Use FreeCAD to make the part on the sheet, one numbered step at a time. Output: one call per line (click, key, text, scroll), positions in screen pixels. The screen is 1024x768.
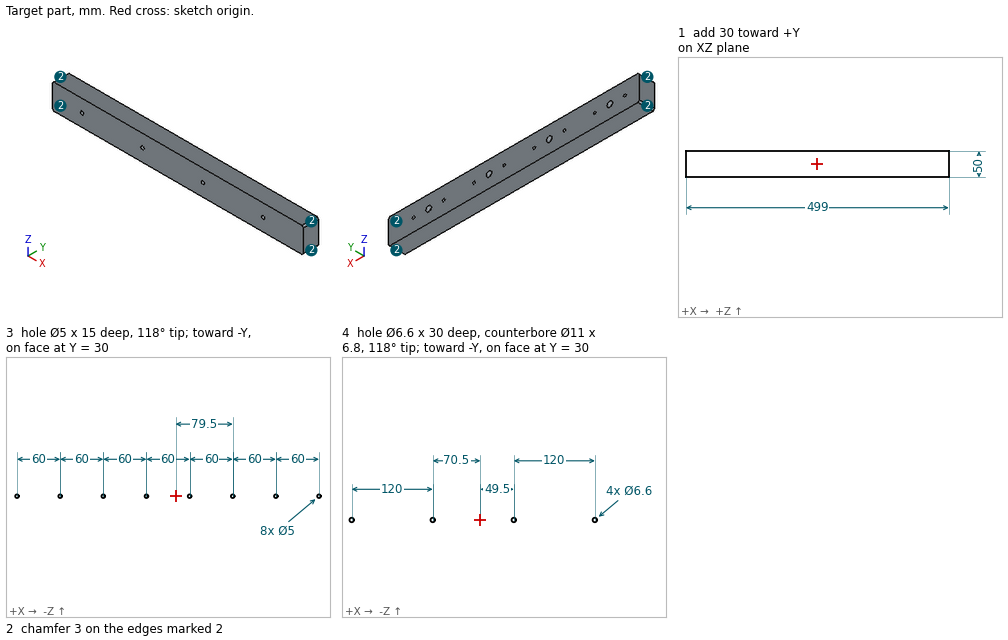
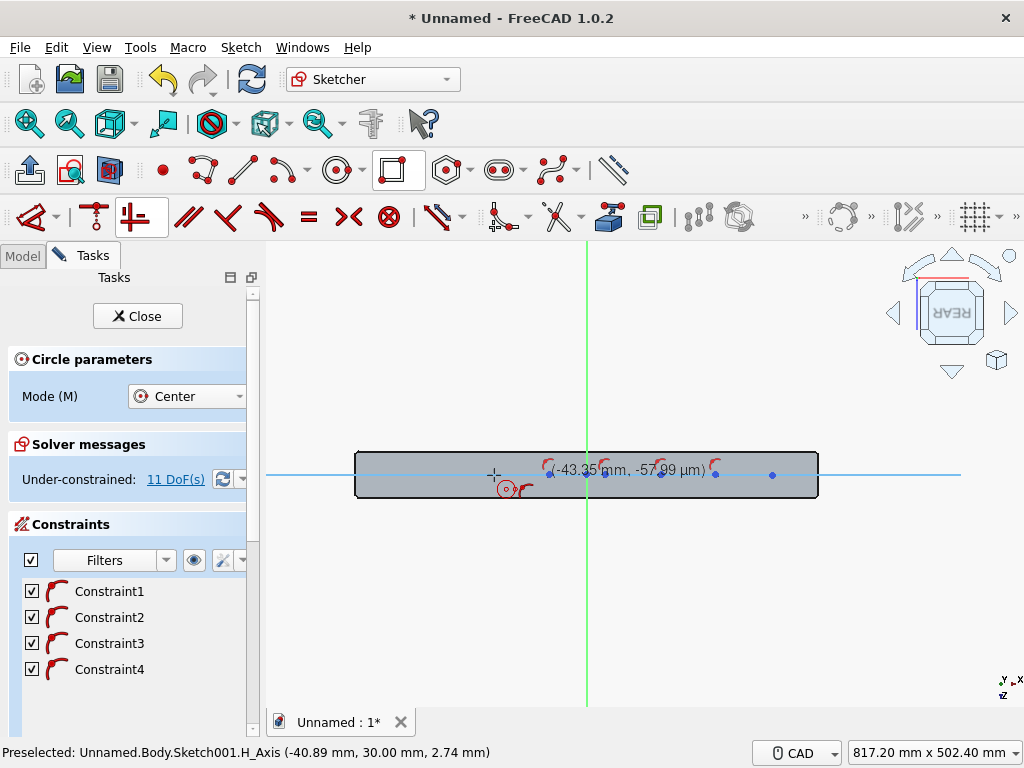
click(494, 475)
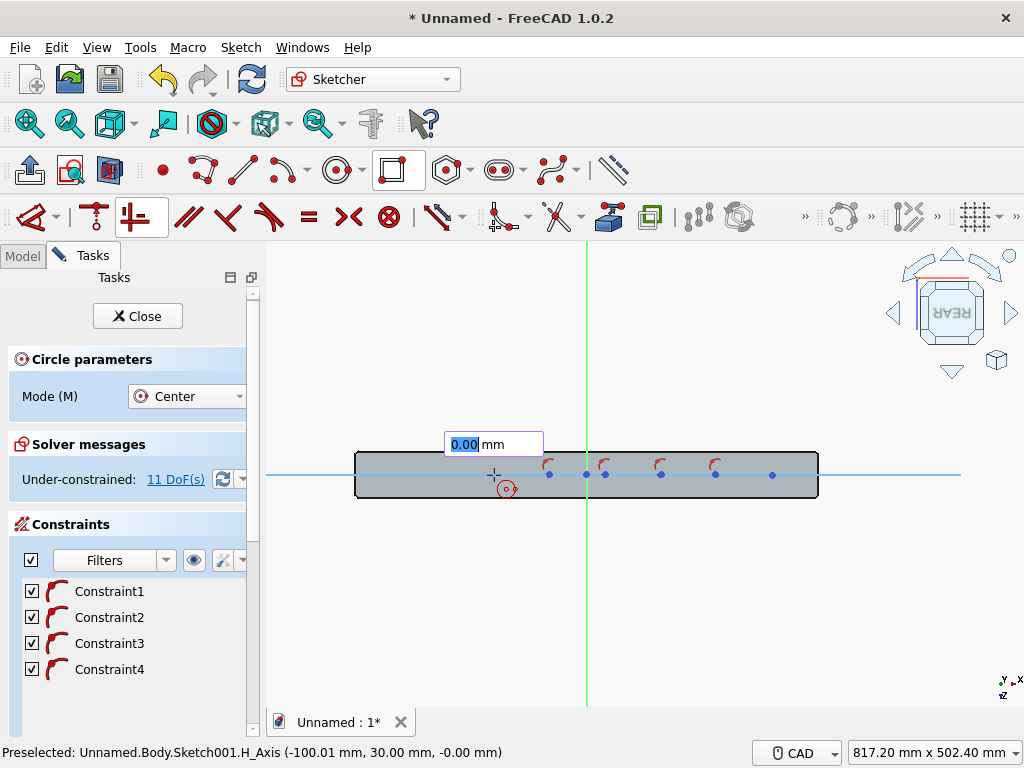
scroll(493, 477, up, 10)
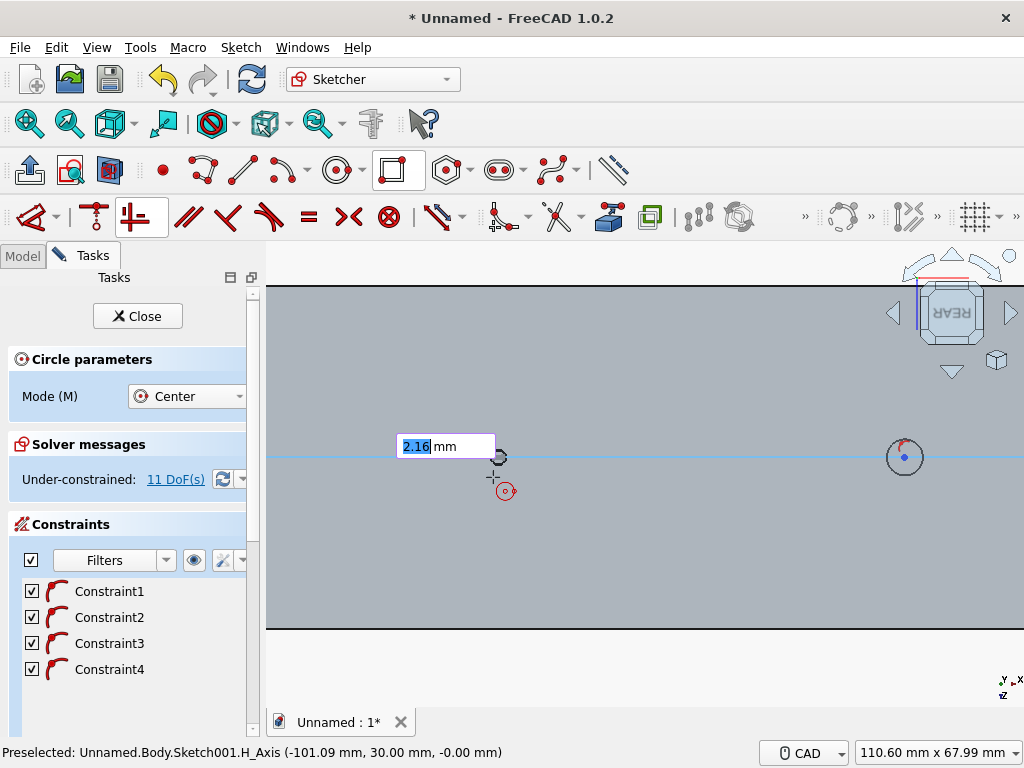
click(489, 474)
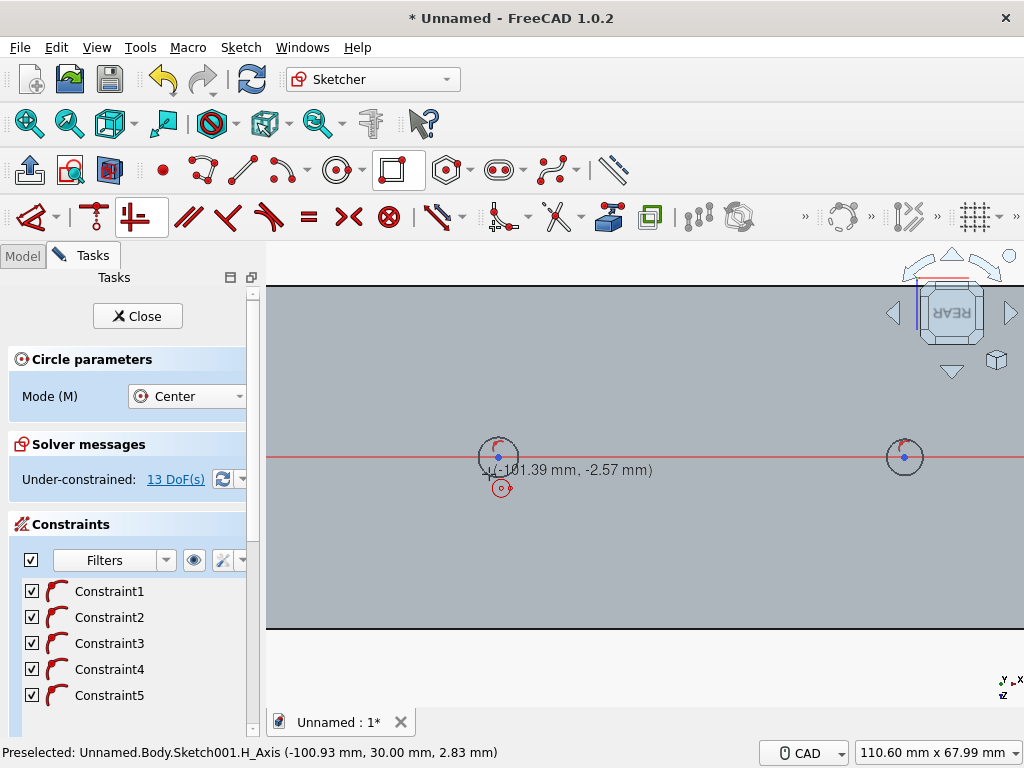
scroll(493, 477, down, 10)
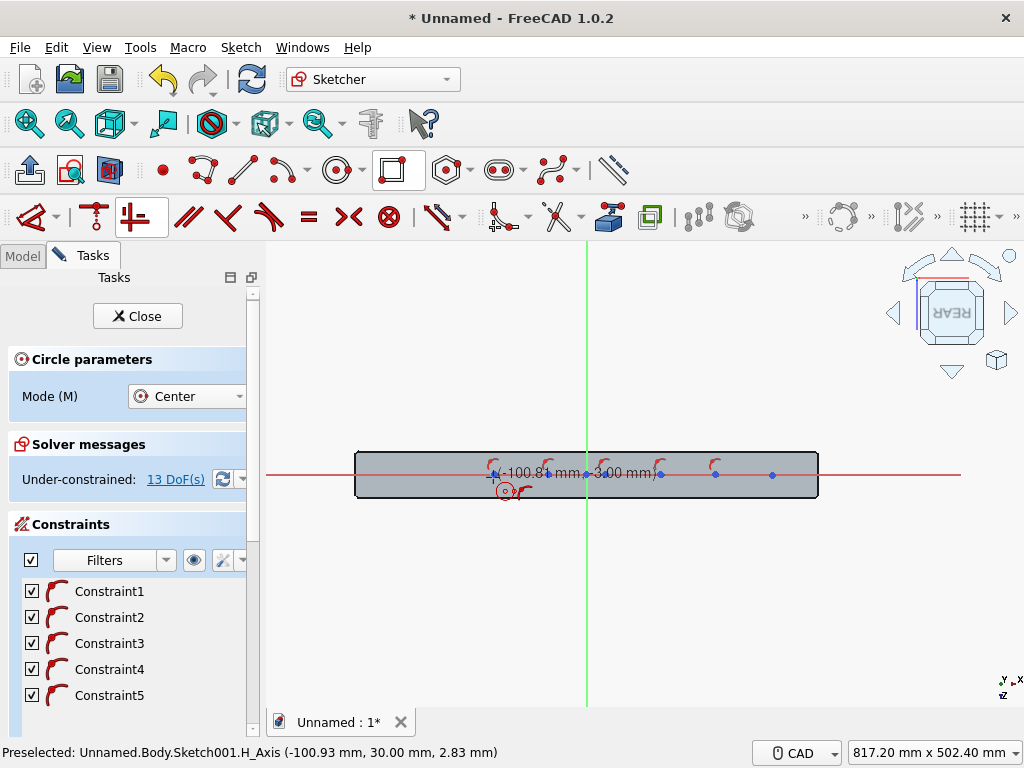
scroll(438, 475, up, 12)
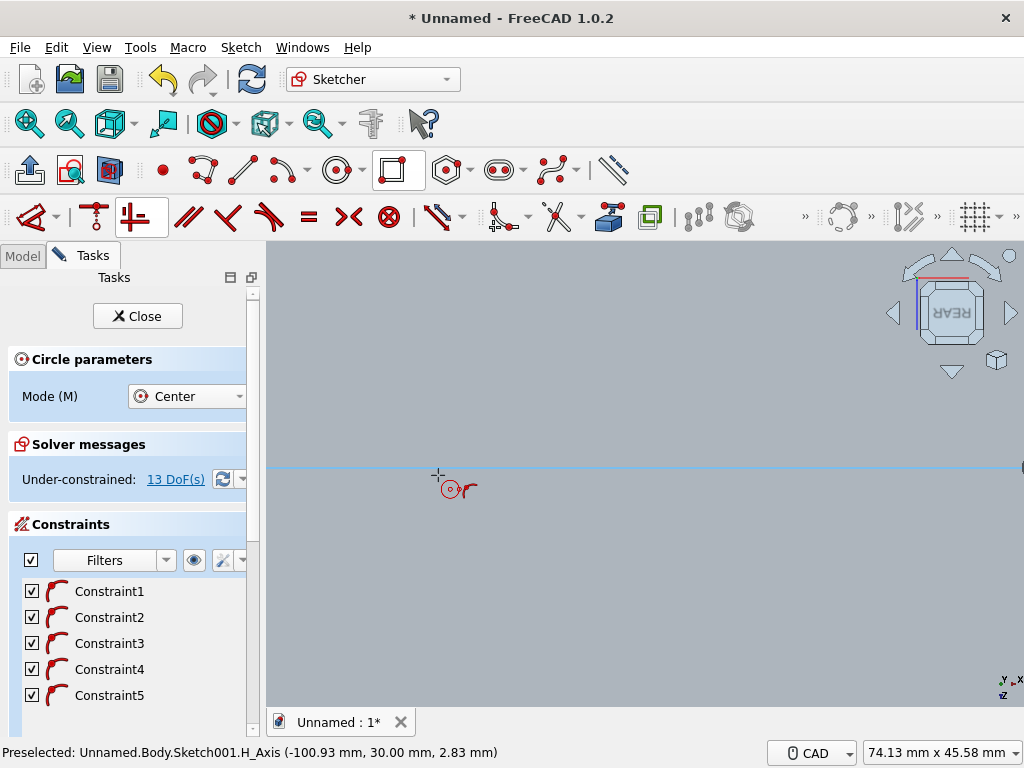
scroll(438, 475, down, 12)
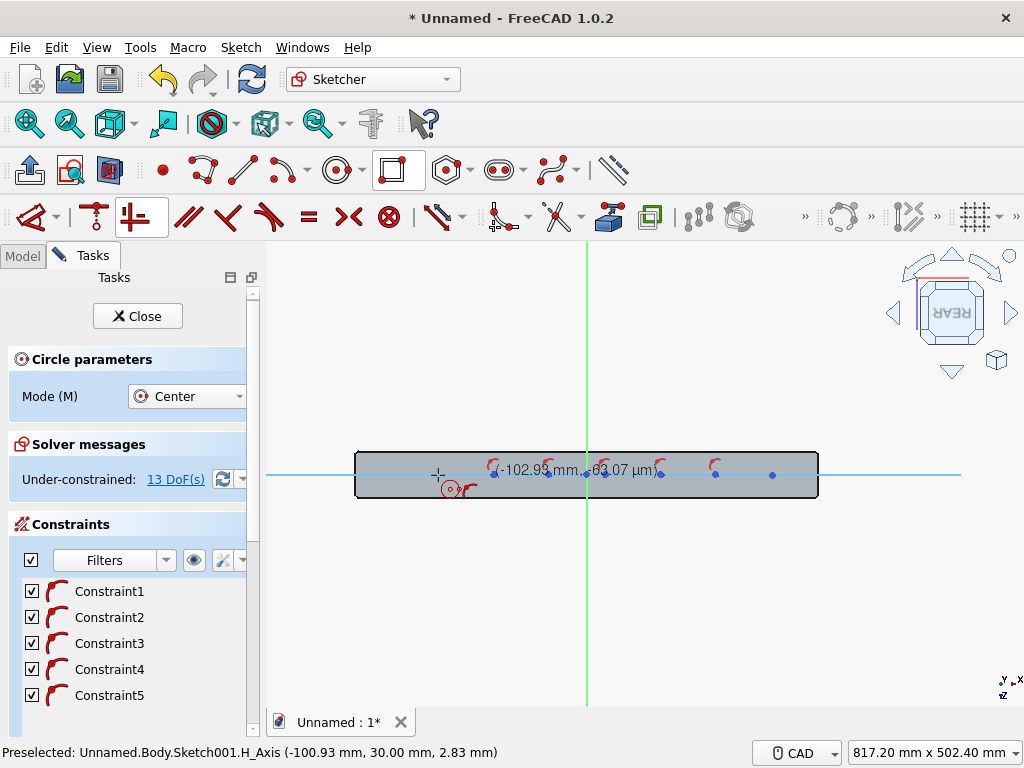
click(438, 475)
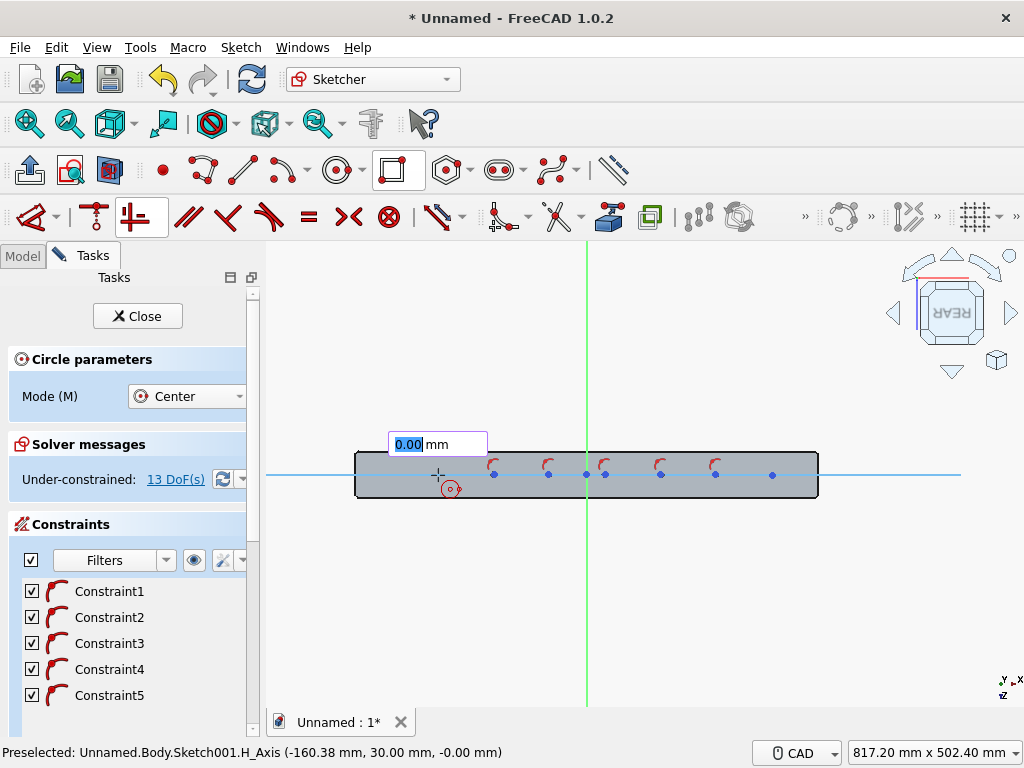
scroll(437, 477, up, 10)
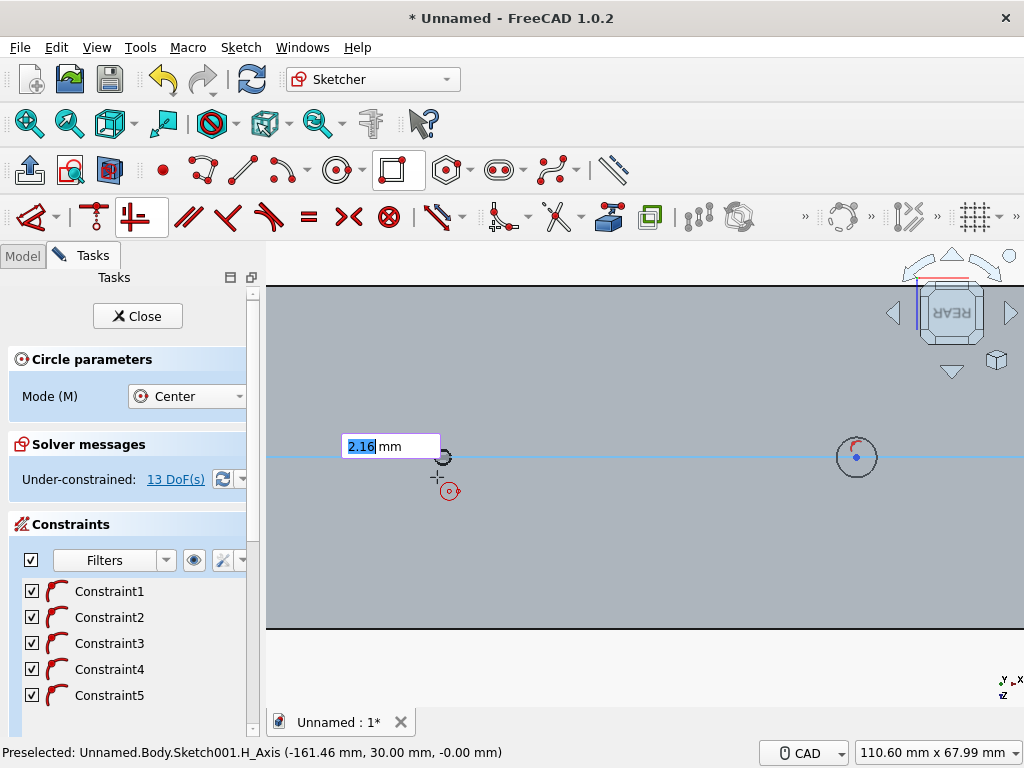
click(436, 474)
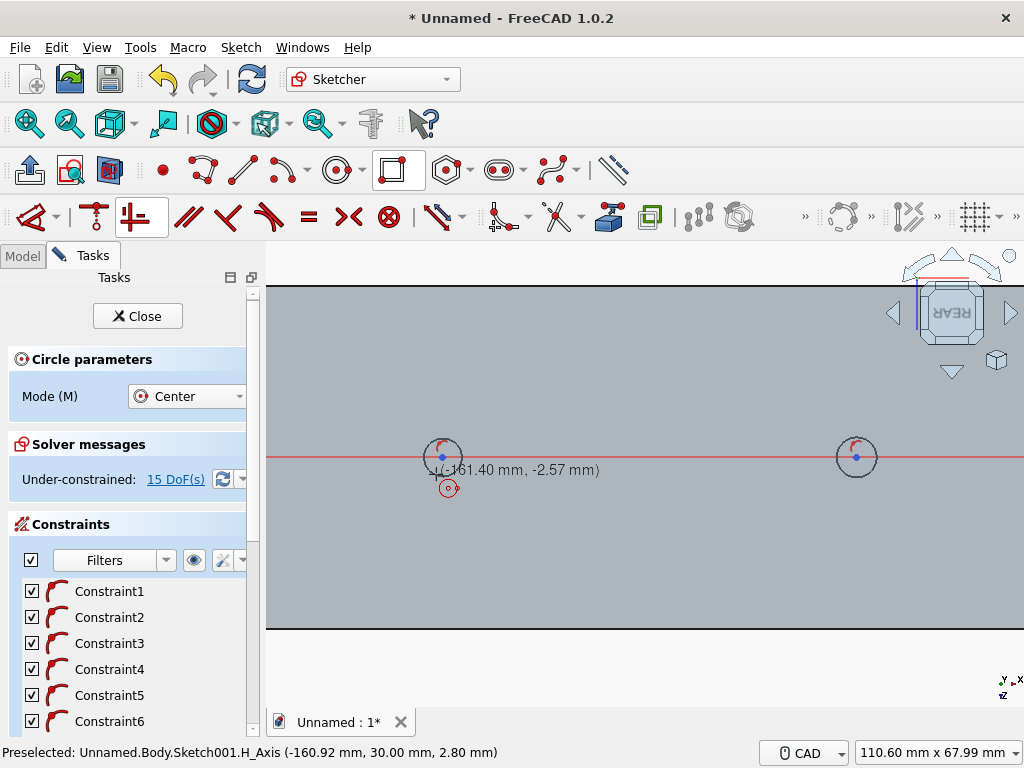
scroll(437, 477, down, 10)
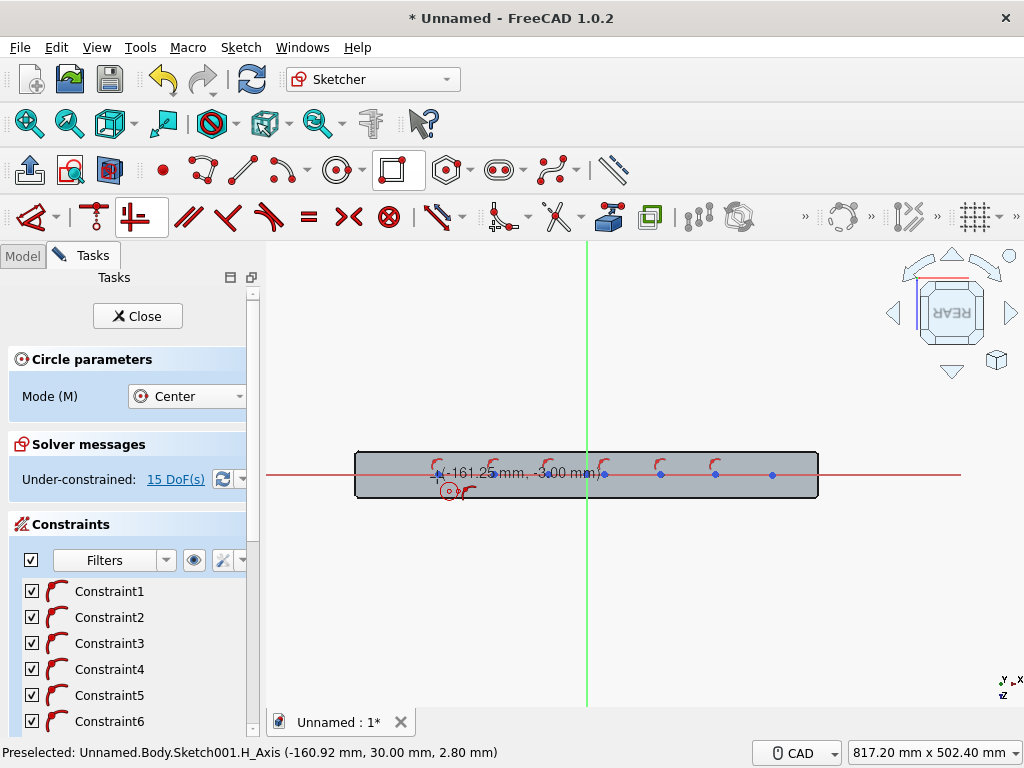
scroll(382, 475, up, 12)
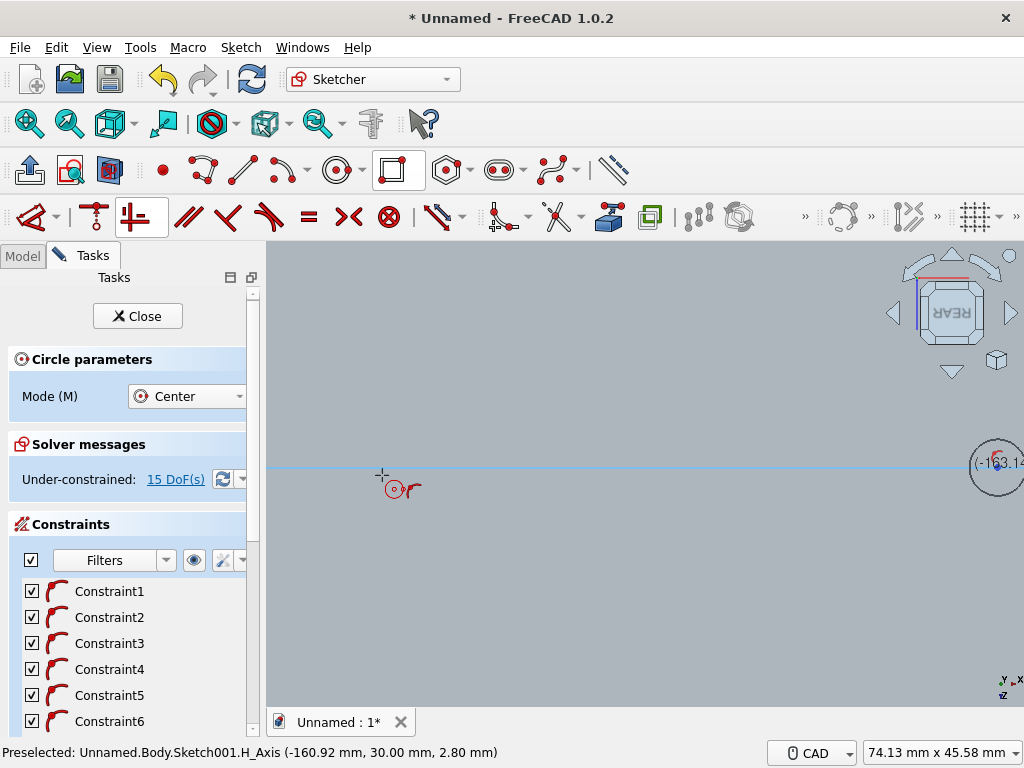
scroll(382, 475, down, 12)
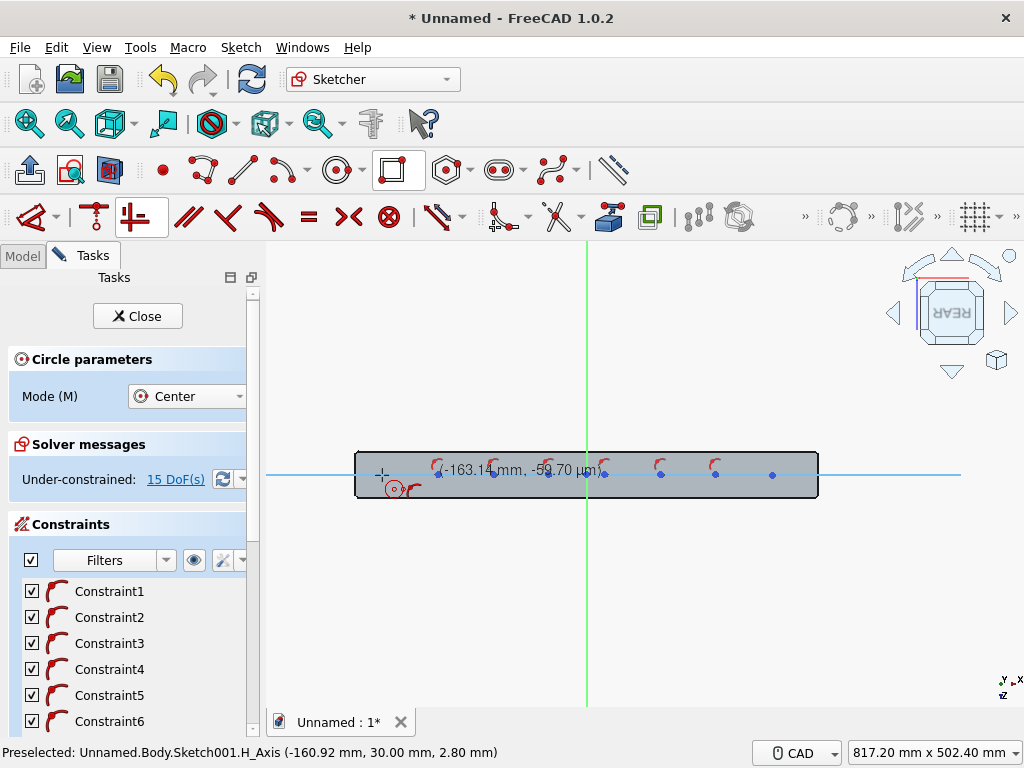
click(382, 475)